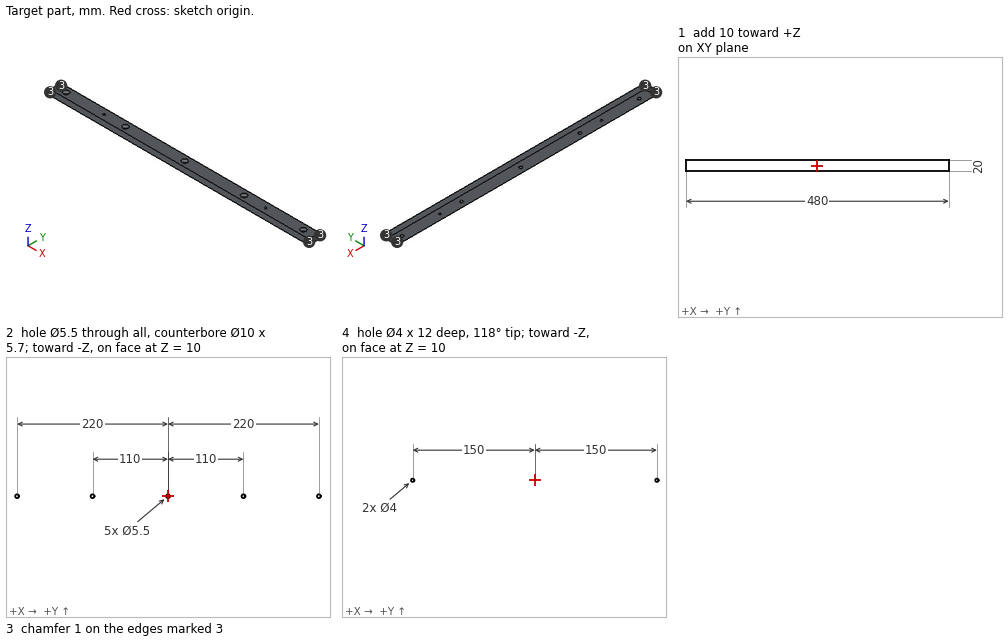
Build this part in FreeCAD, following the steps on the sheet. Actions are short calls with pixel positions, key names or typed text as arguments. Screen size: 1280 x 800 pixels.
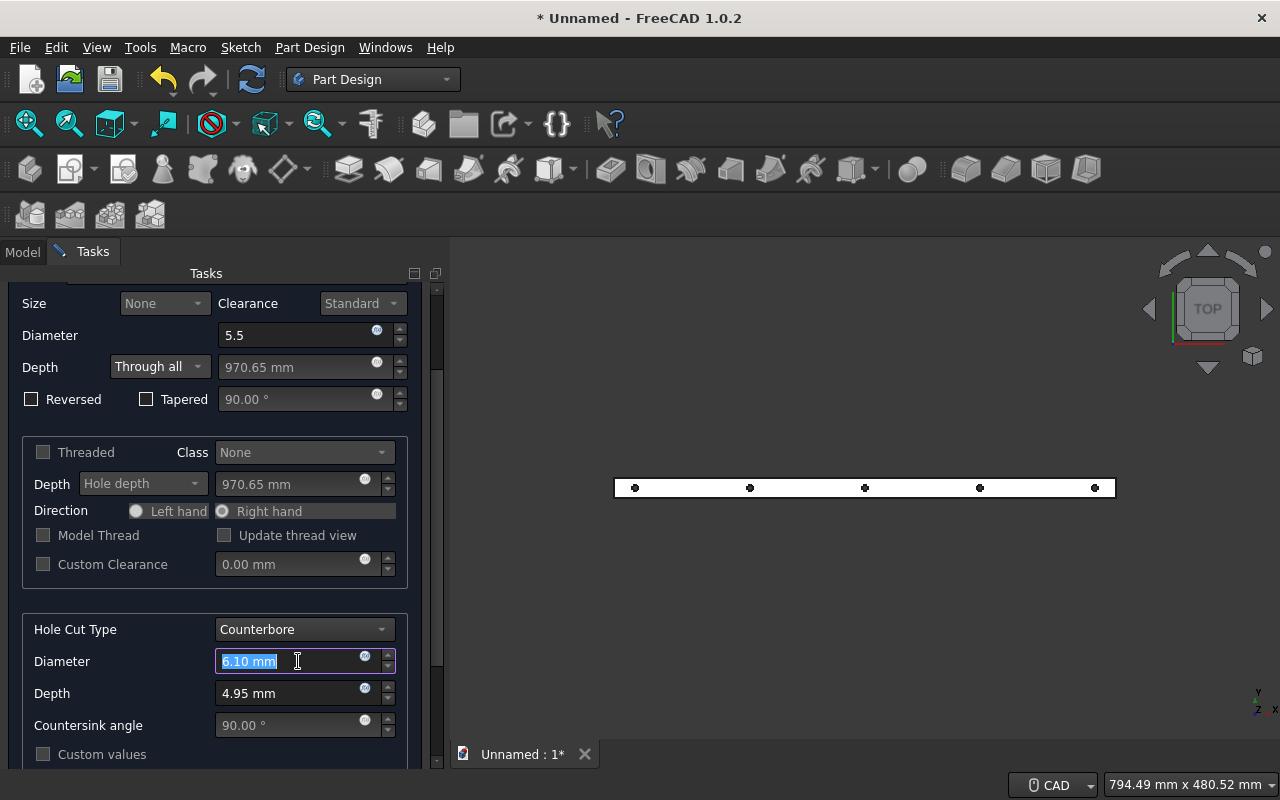
text(10)
key(Tab)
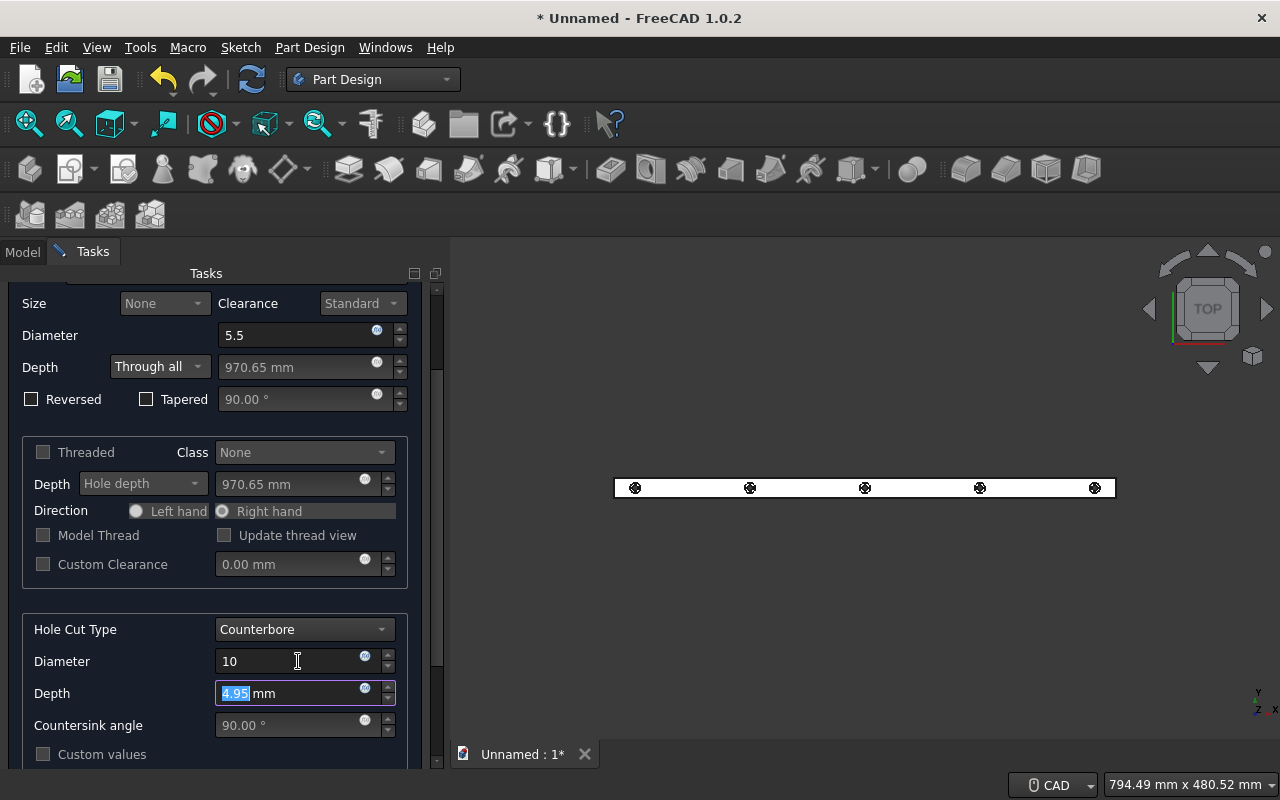
text(5.7)
key(Tab)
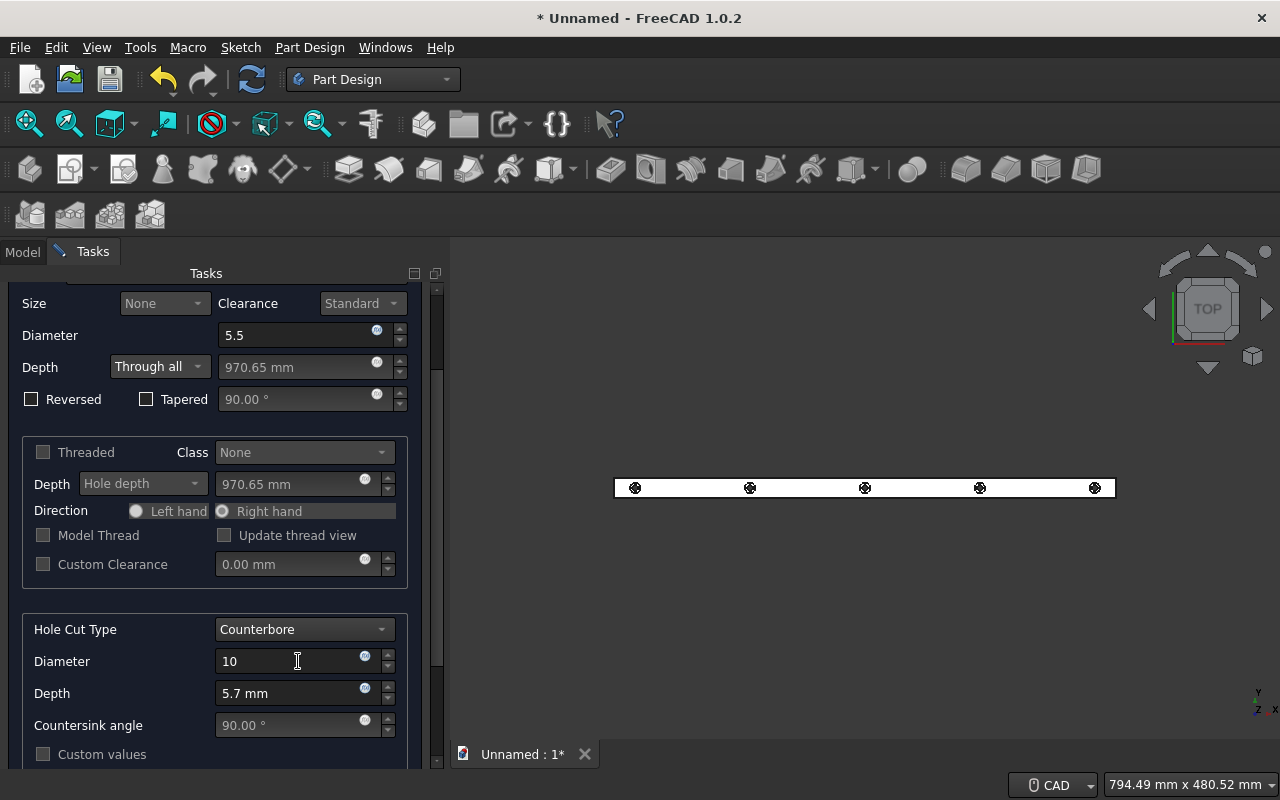
scroll(437, 526, up, 3)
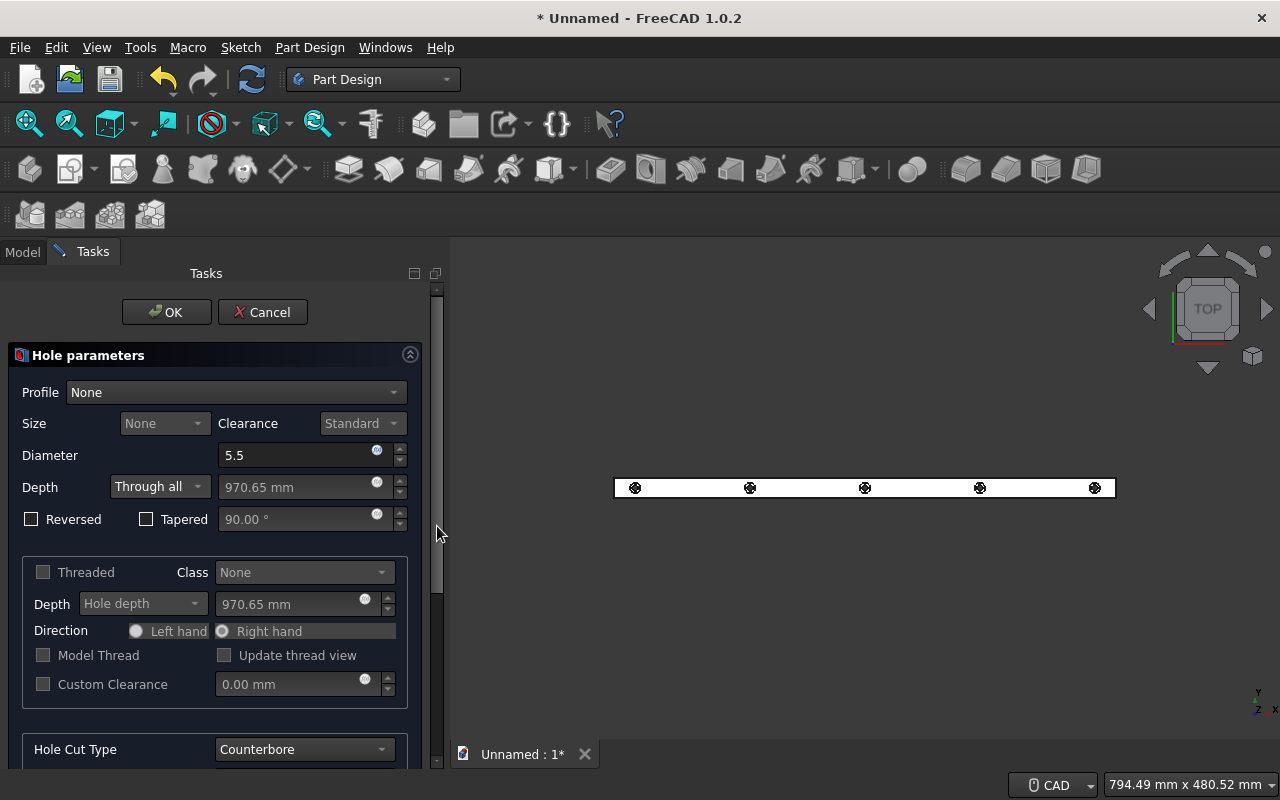
click(167, 312)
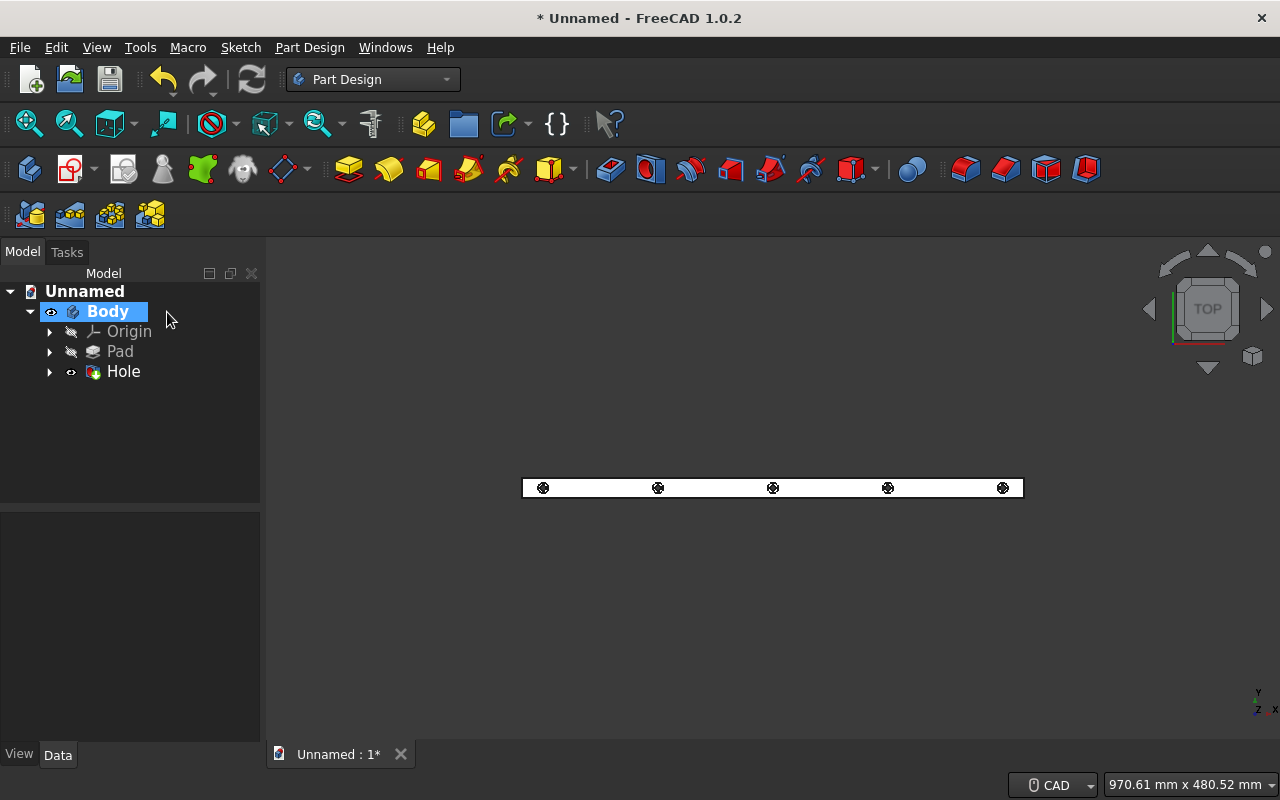
scroll(1024, 497, up, 7)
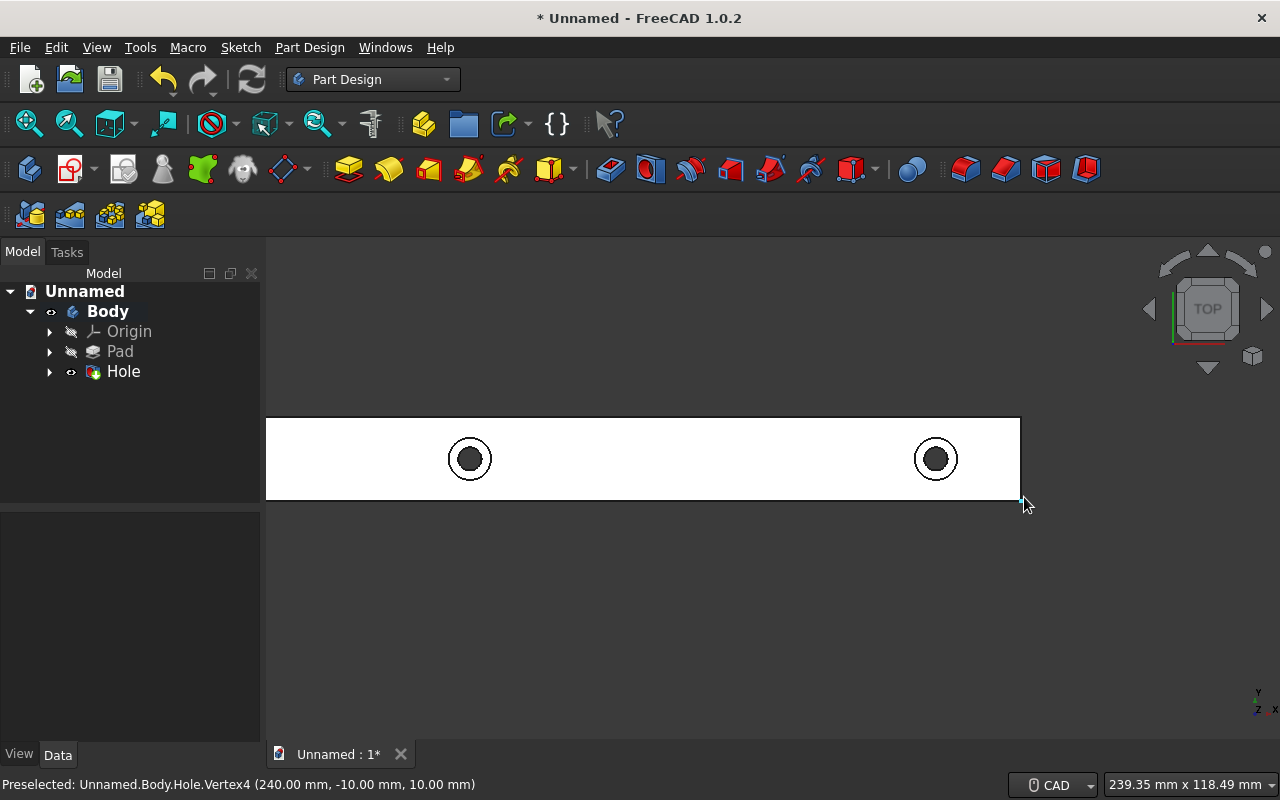
click(30, 124)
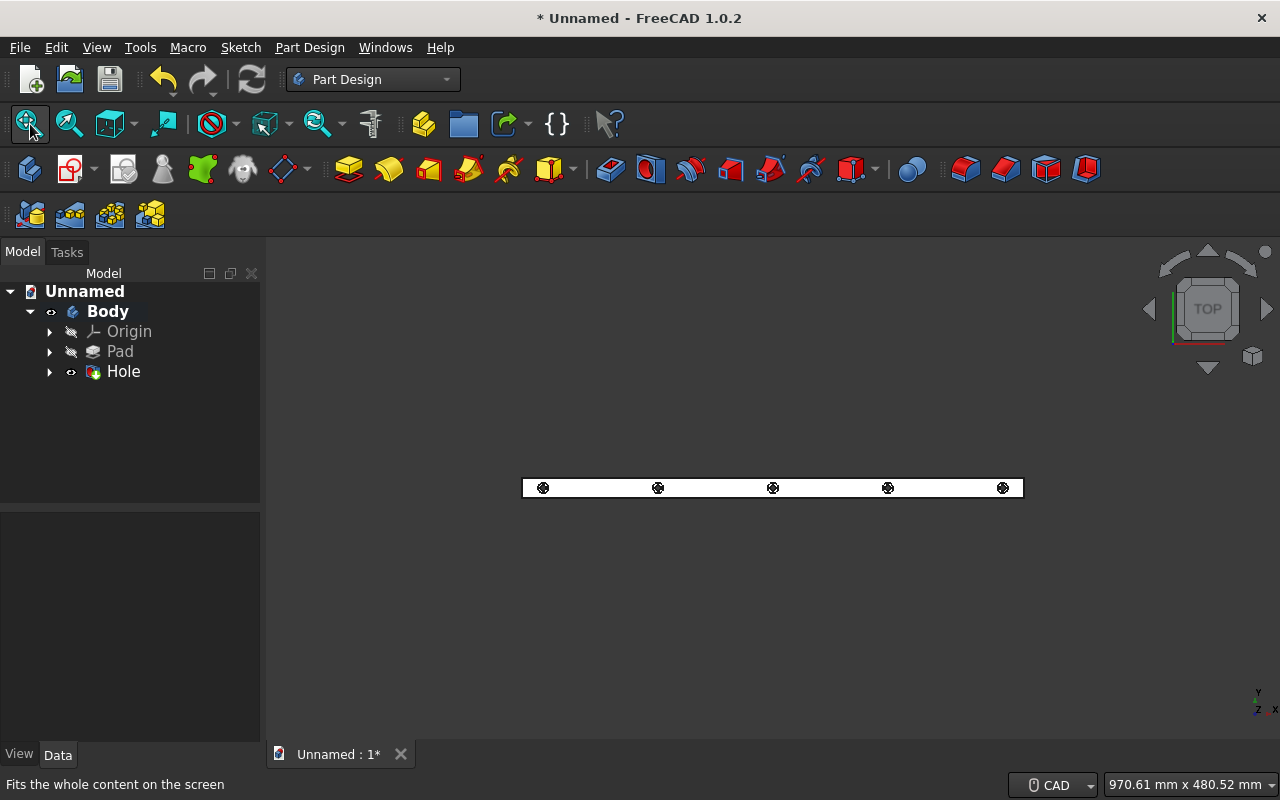
key(0)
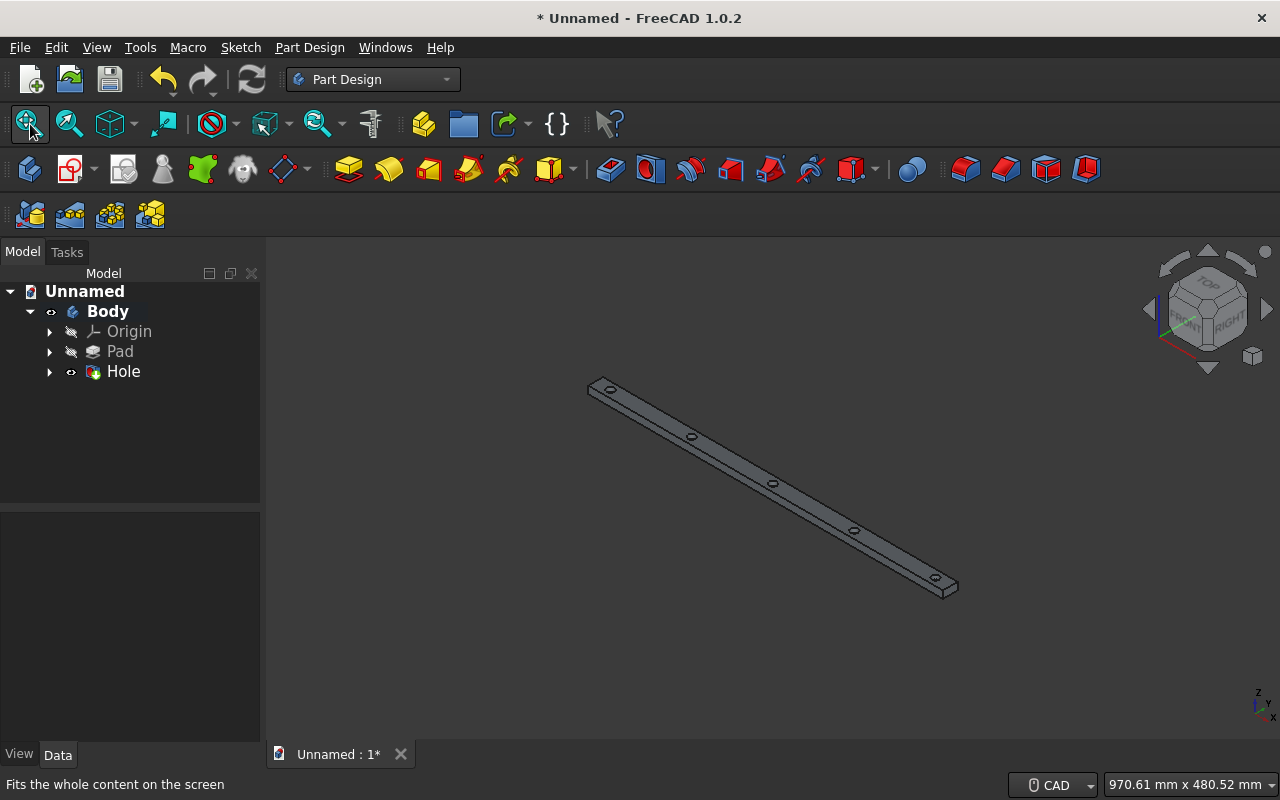
click(30, 124)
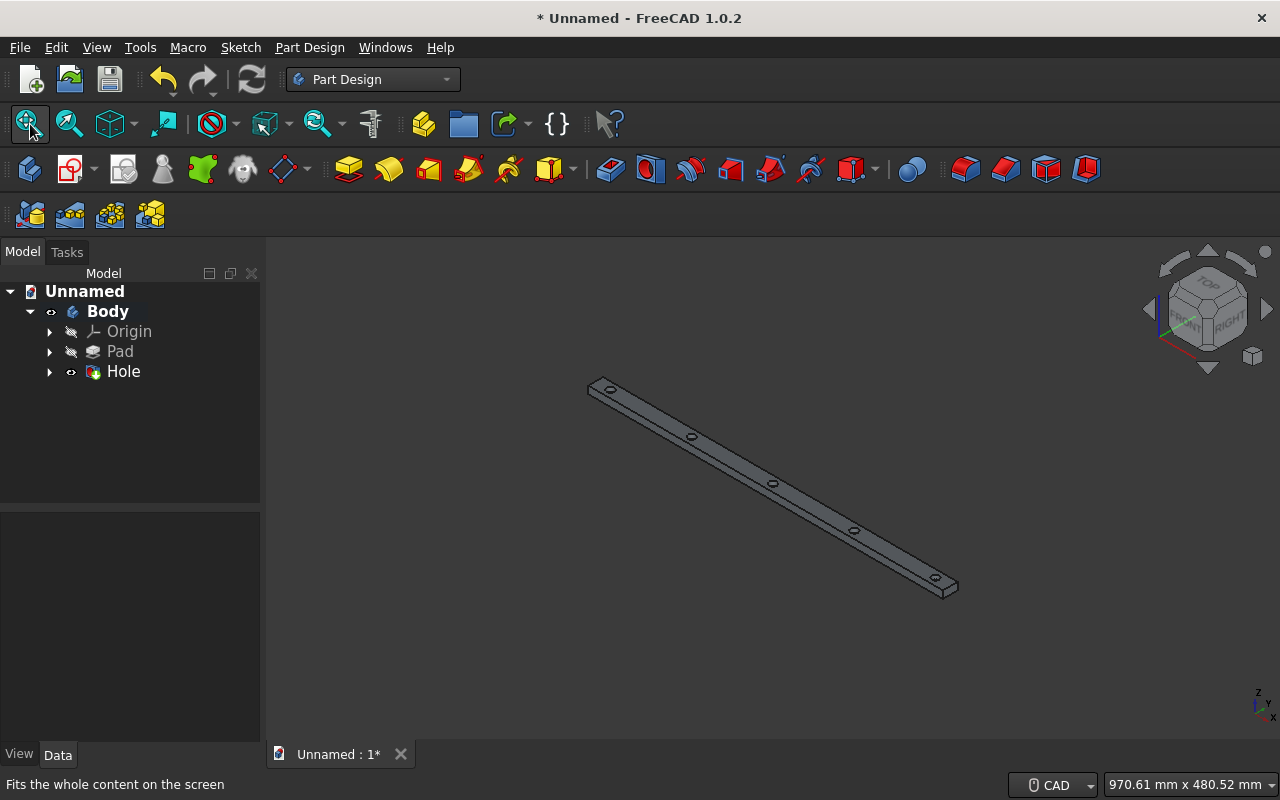
click(943, 596)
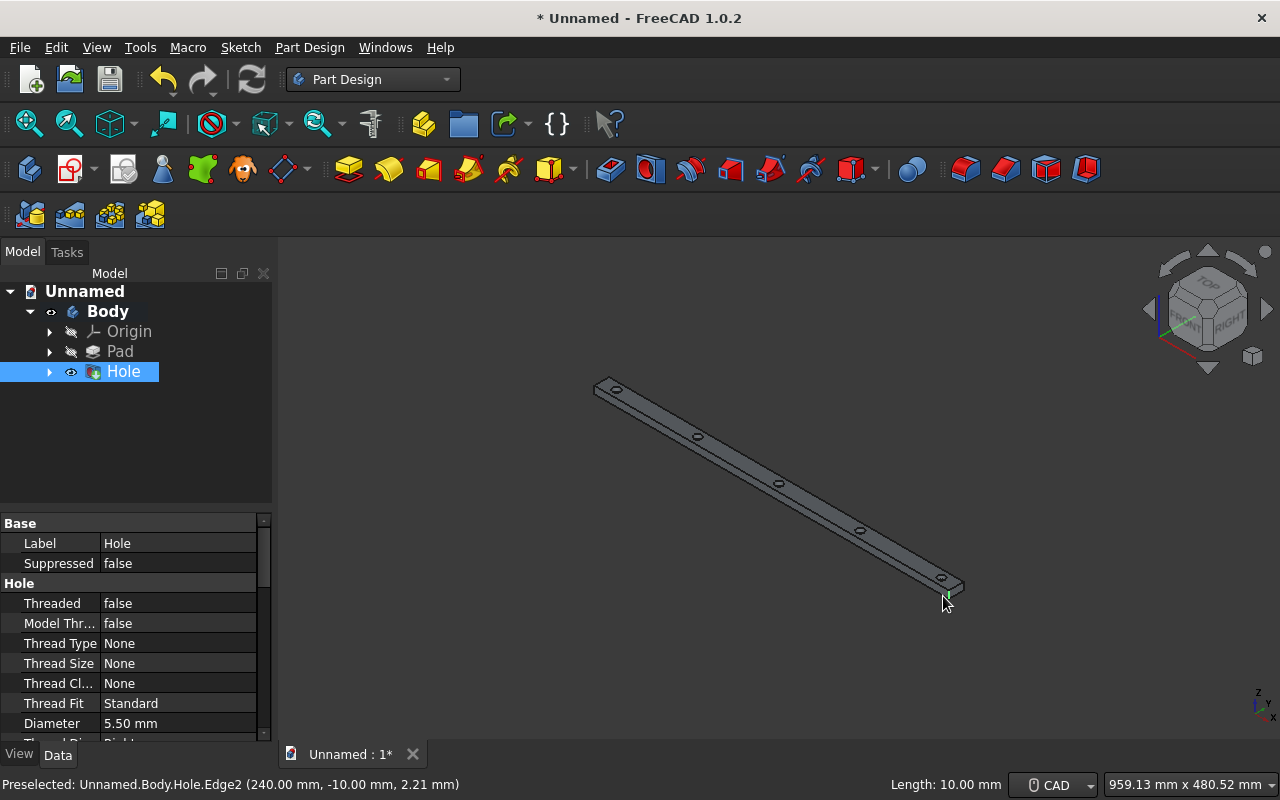
scroll(594, 389, up, 7)